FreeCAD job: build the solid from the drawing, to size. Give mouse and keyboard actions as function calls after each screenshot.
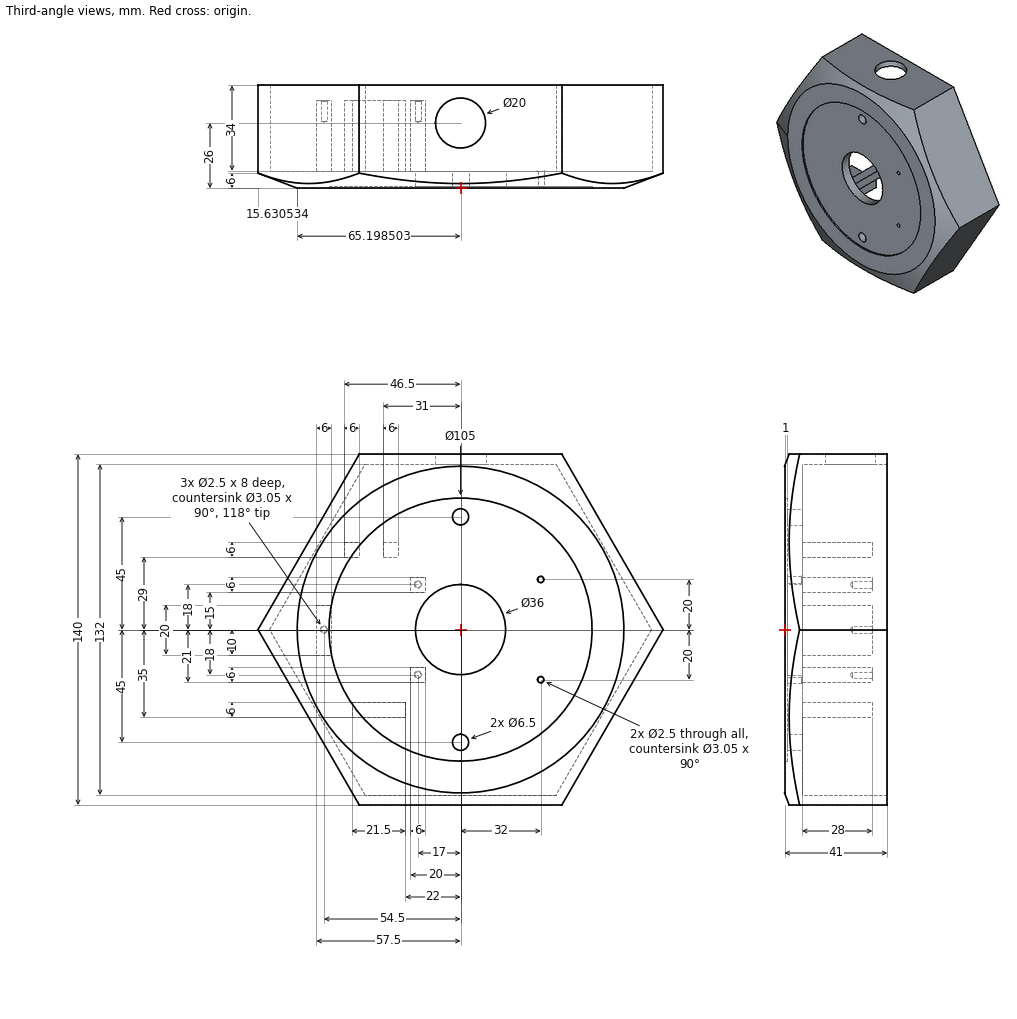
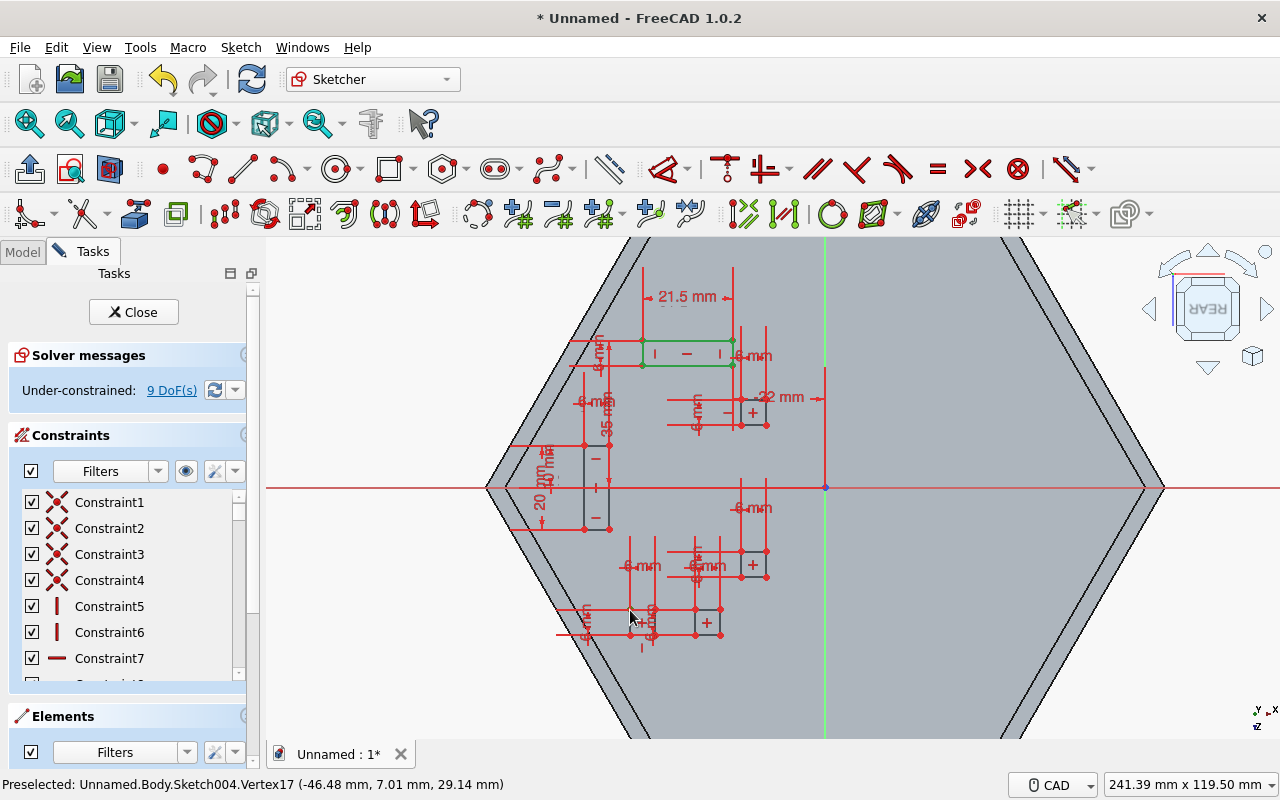
click(690, 170)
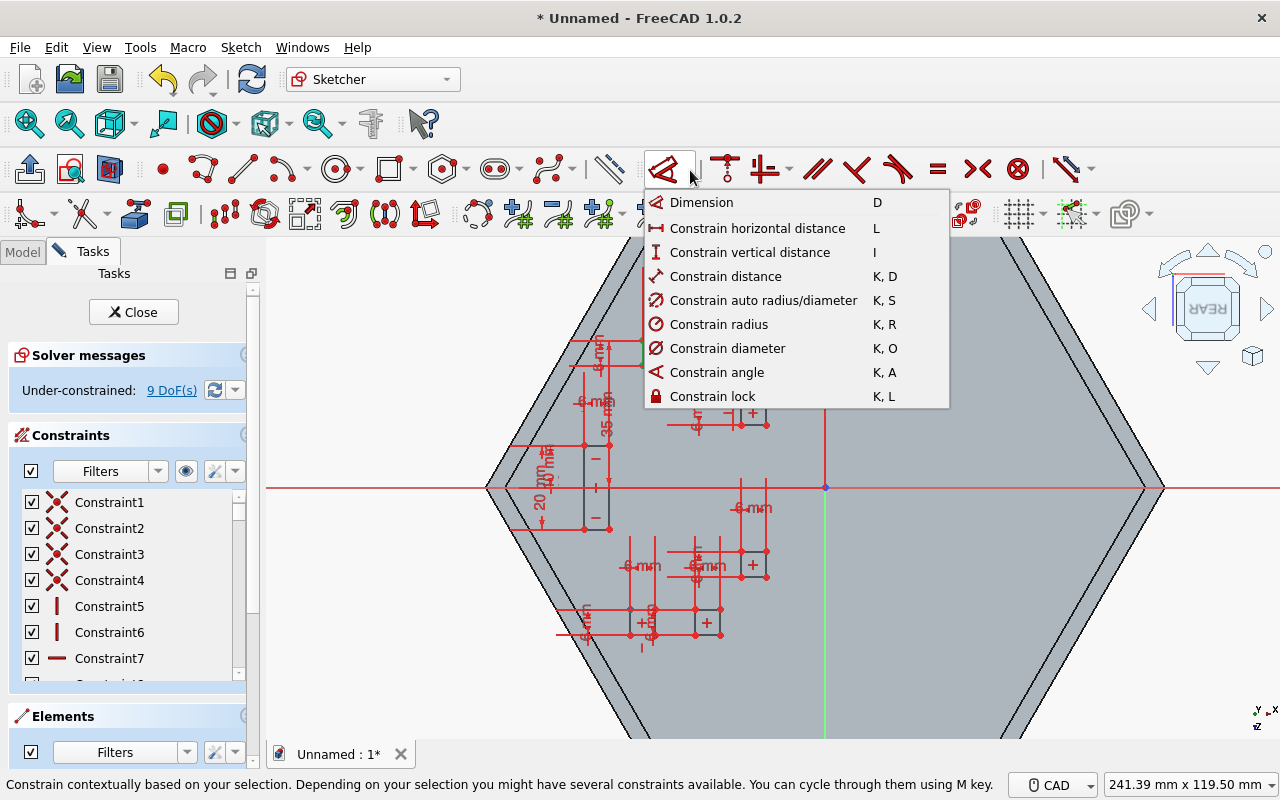
click(797, 252)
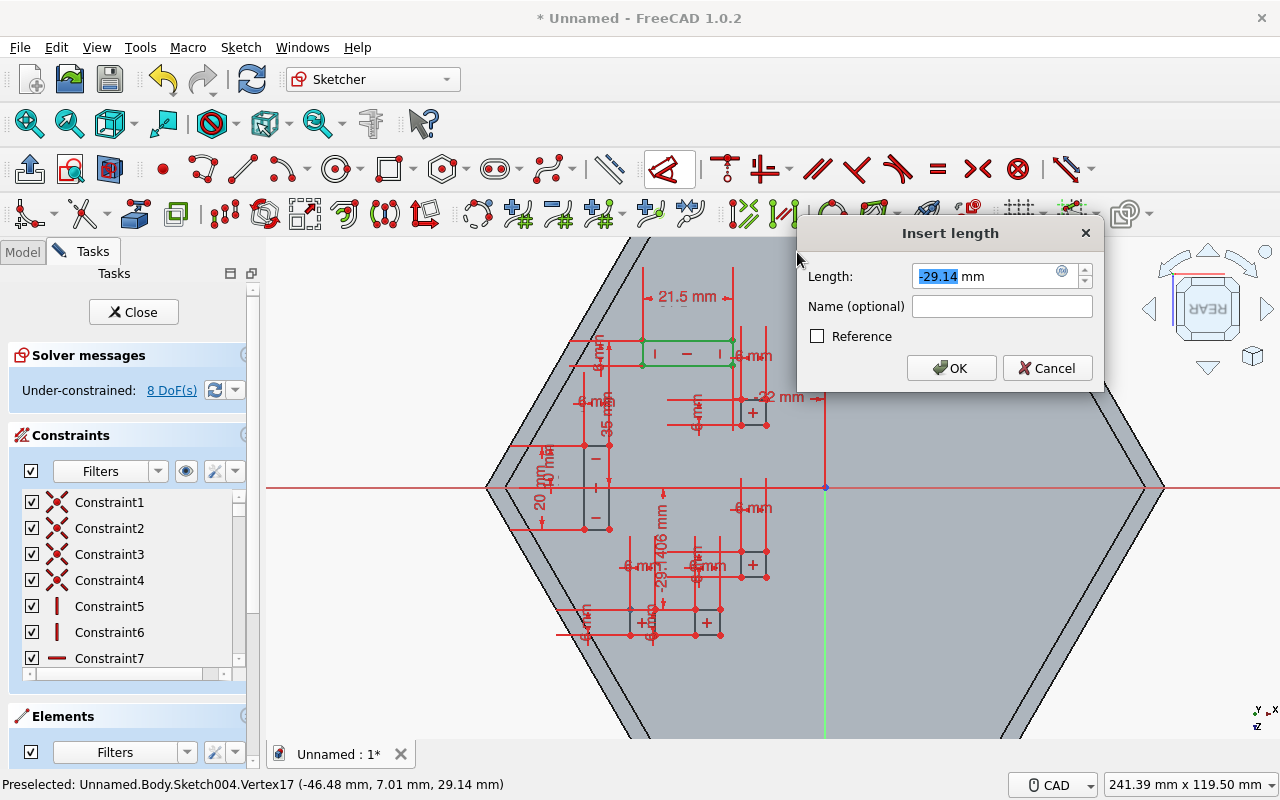
text(-29)
key(Return)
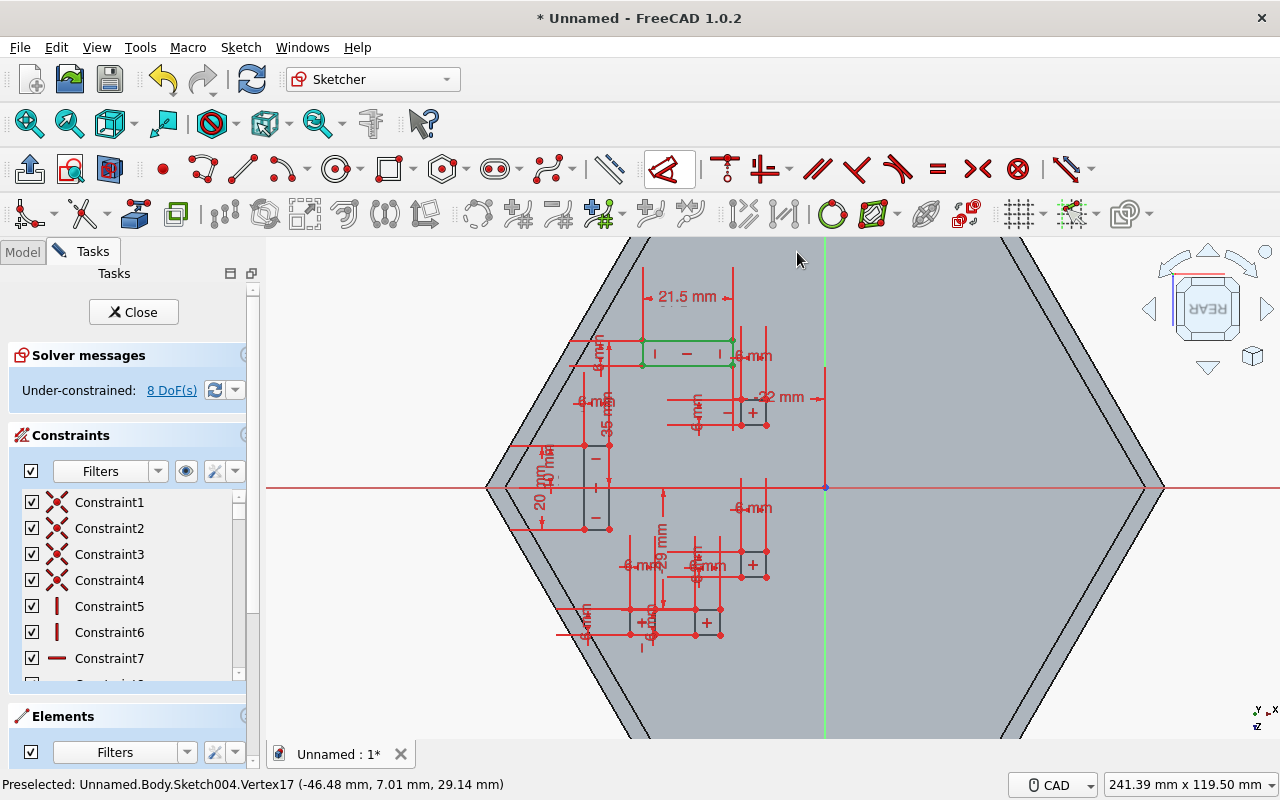
click(695, 610)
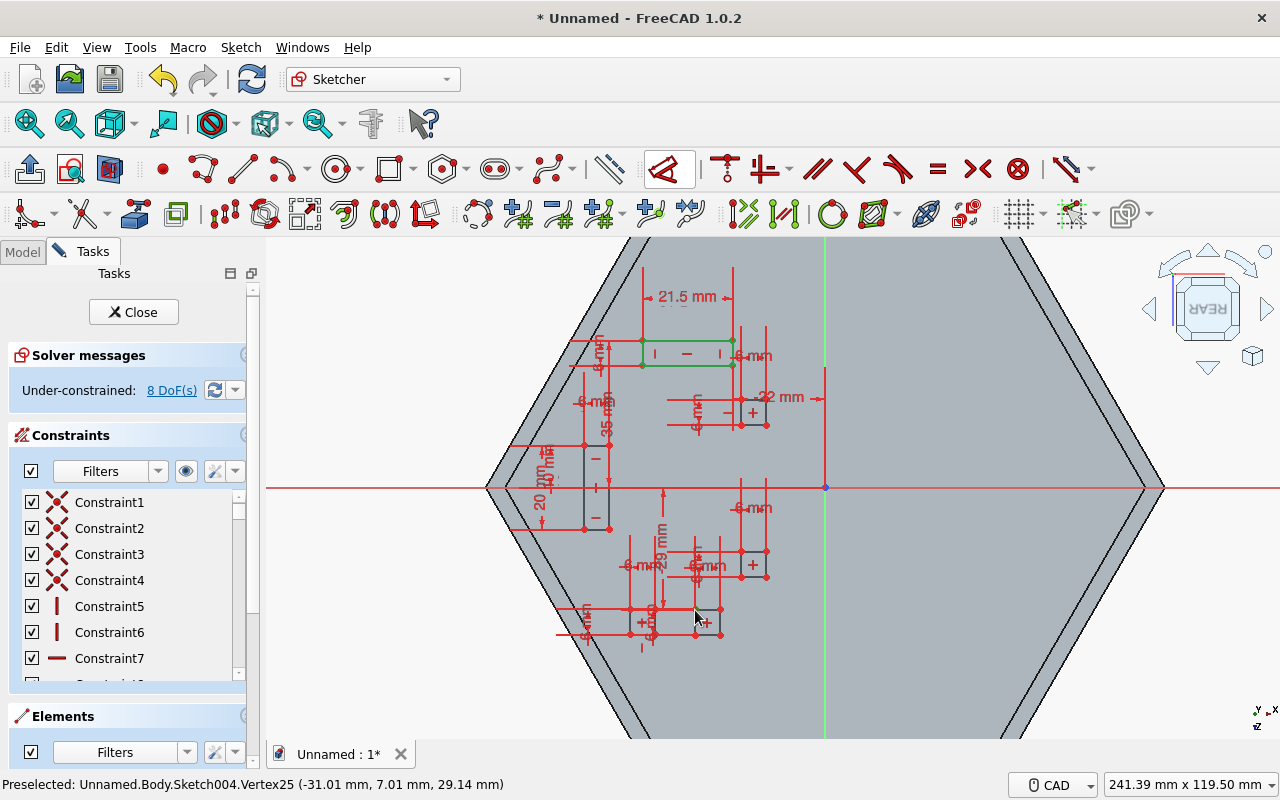
key(l)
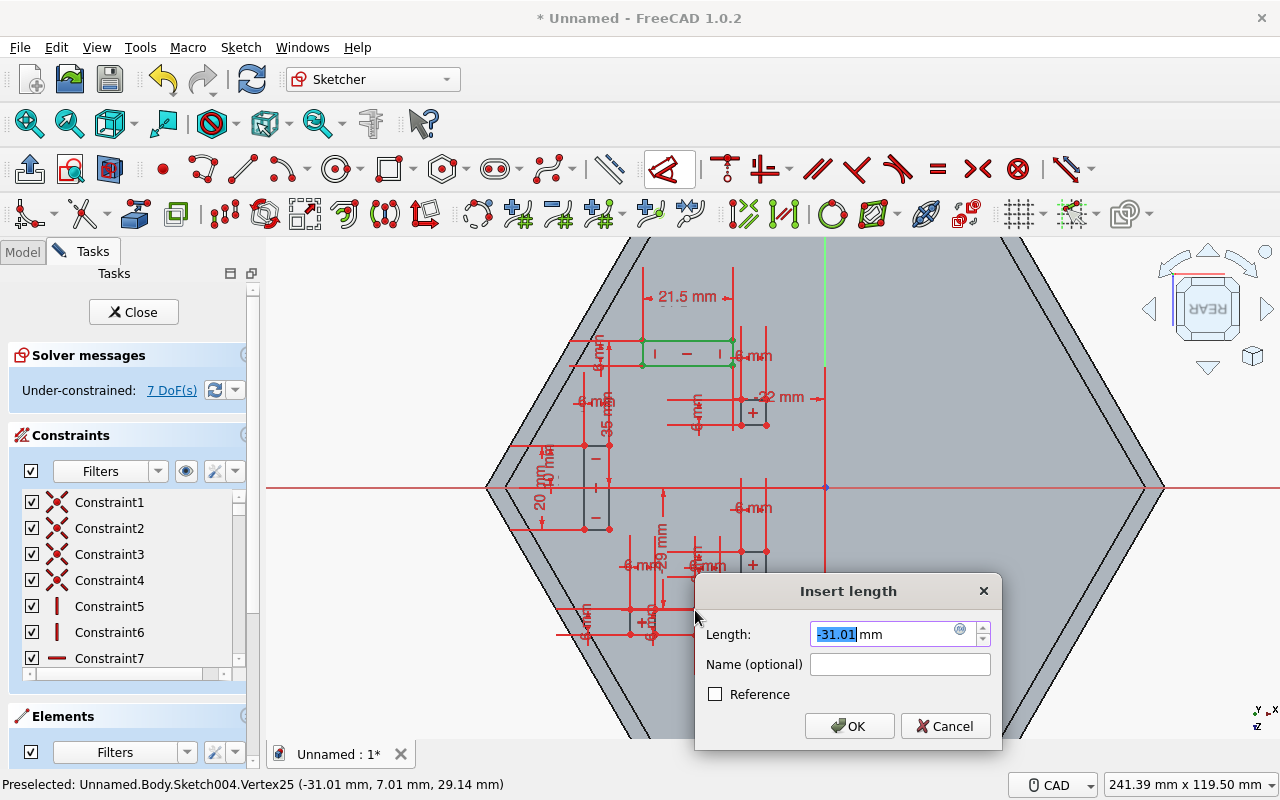
text(-31)
key(Return)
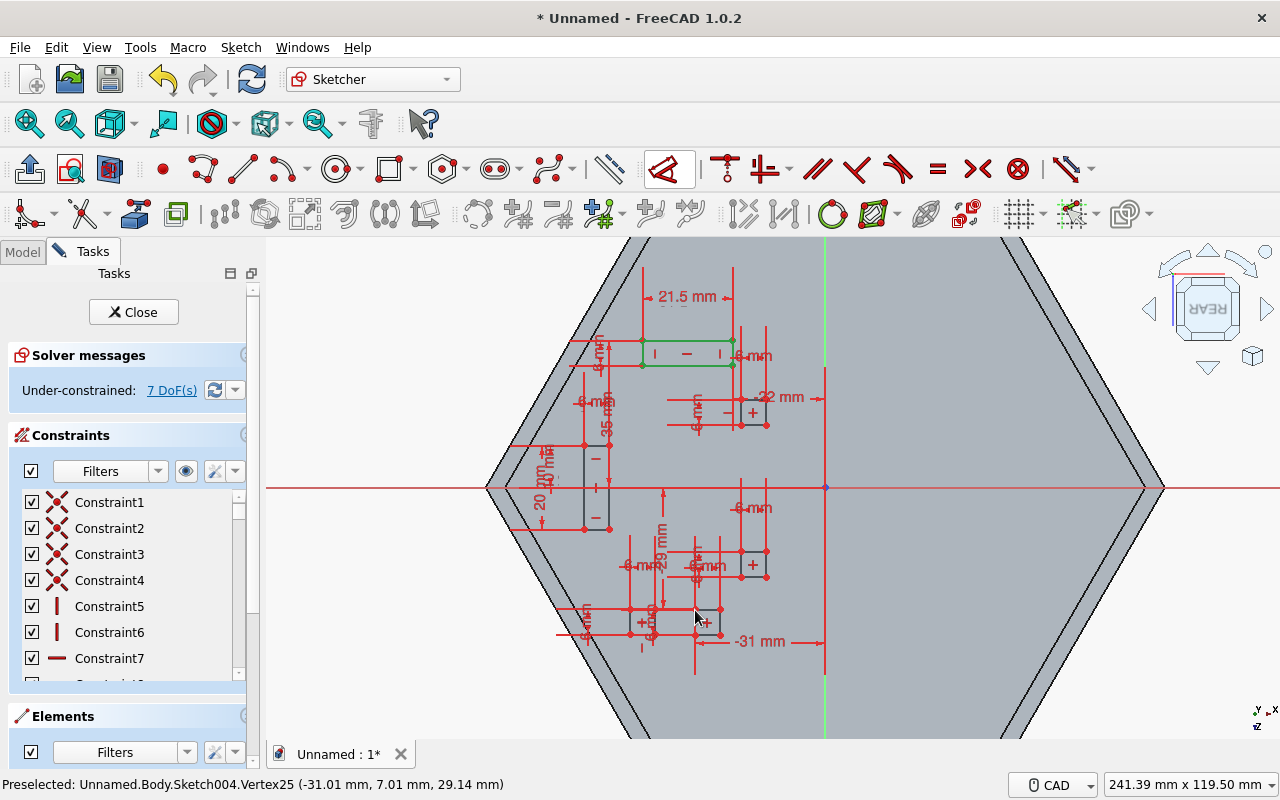
click(695, 610)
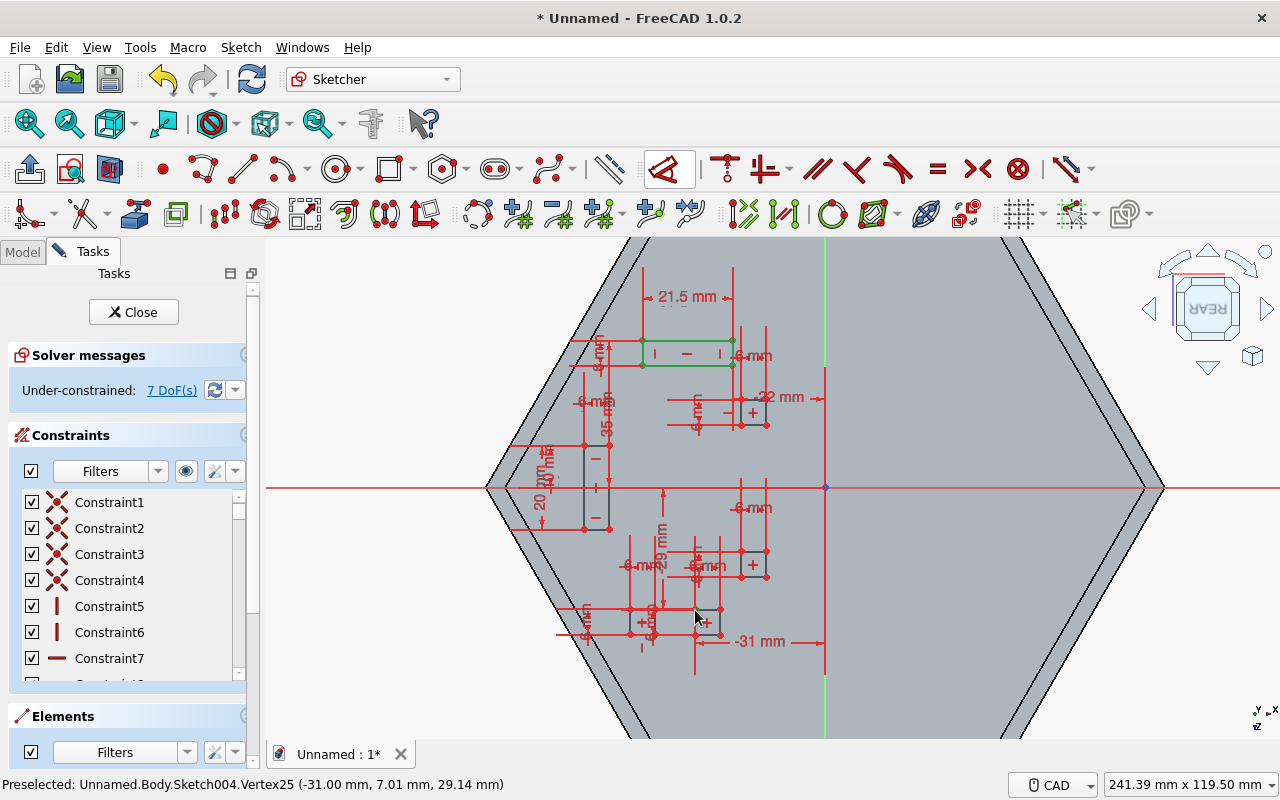
key(i)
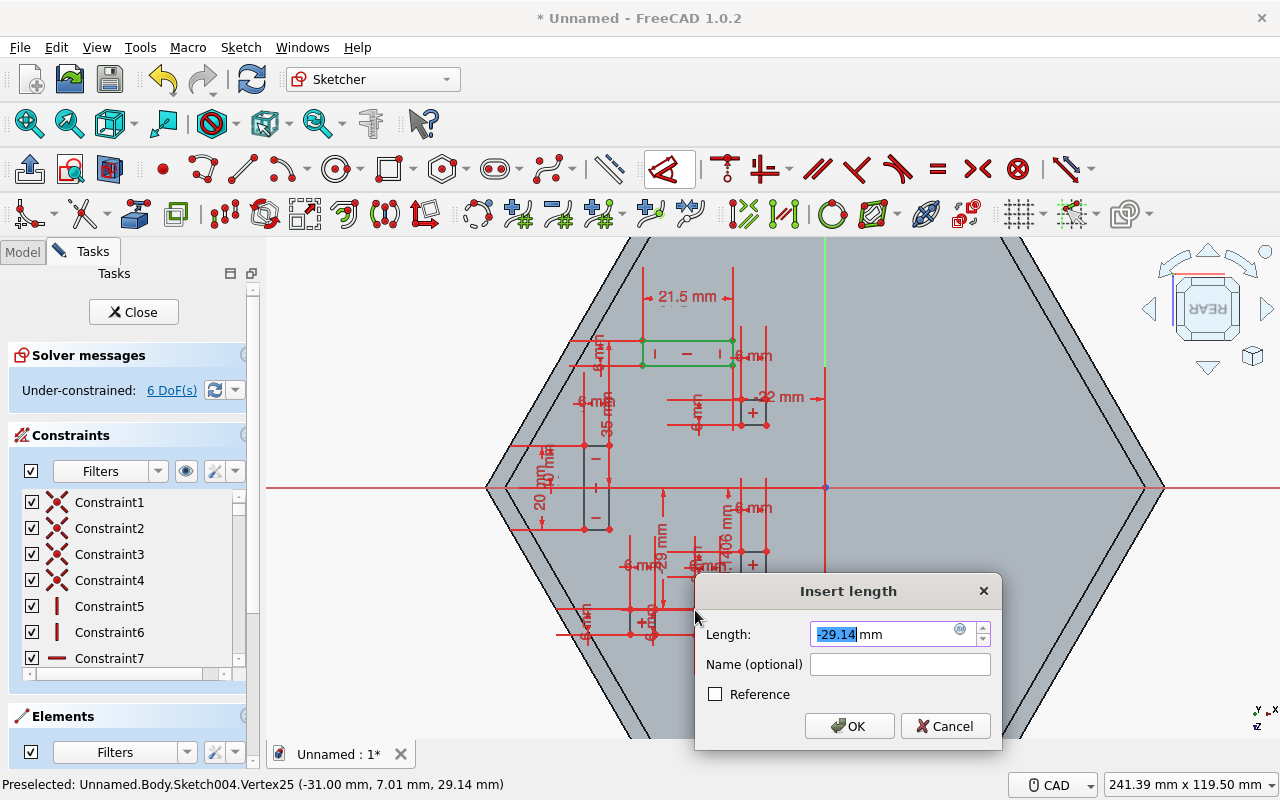
text(-29)
key(Return)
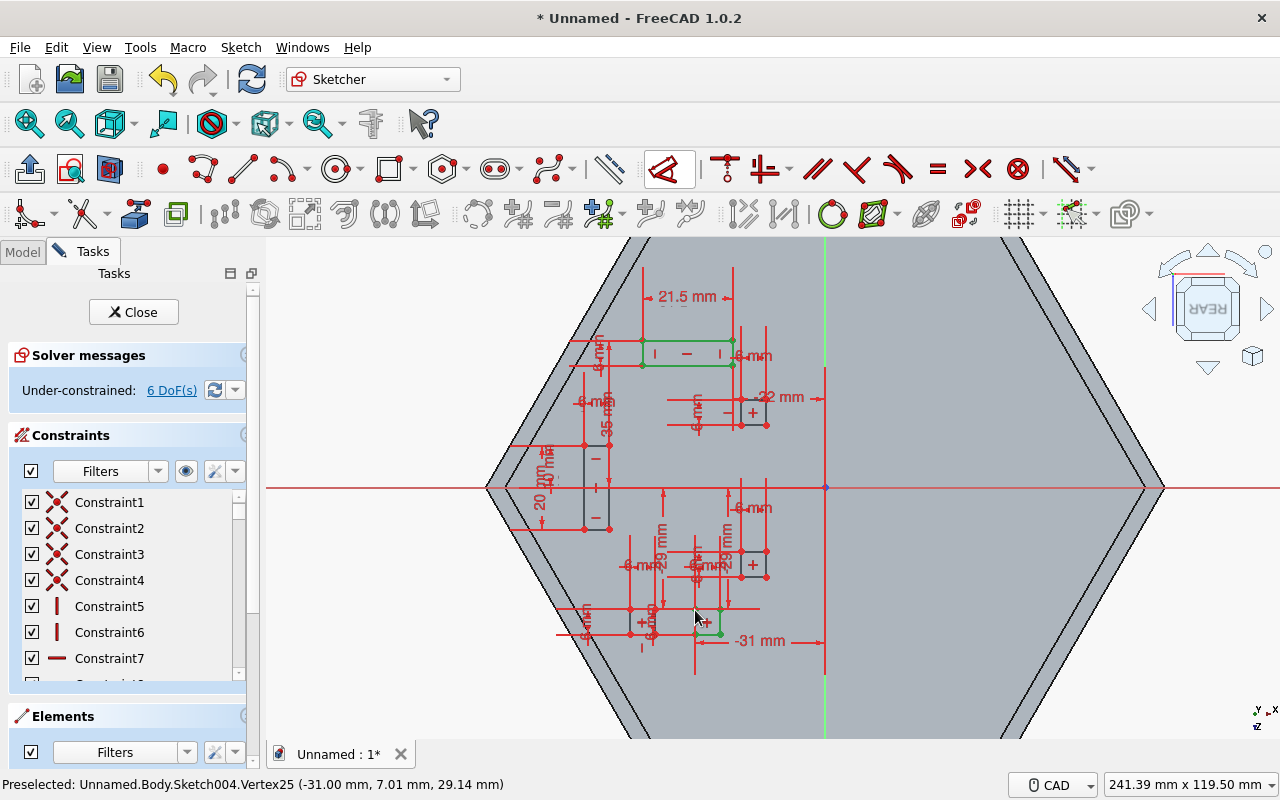
click(741, 400)